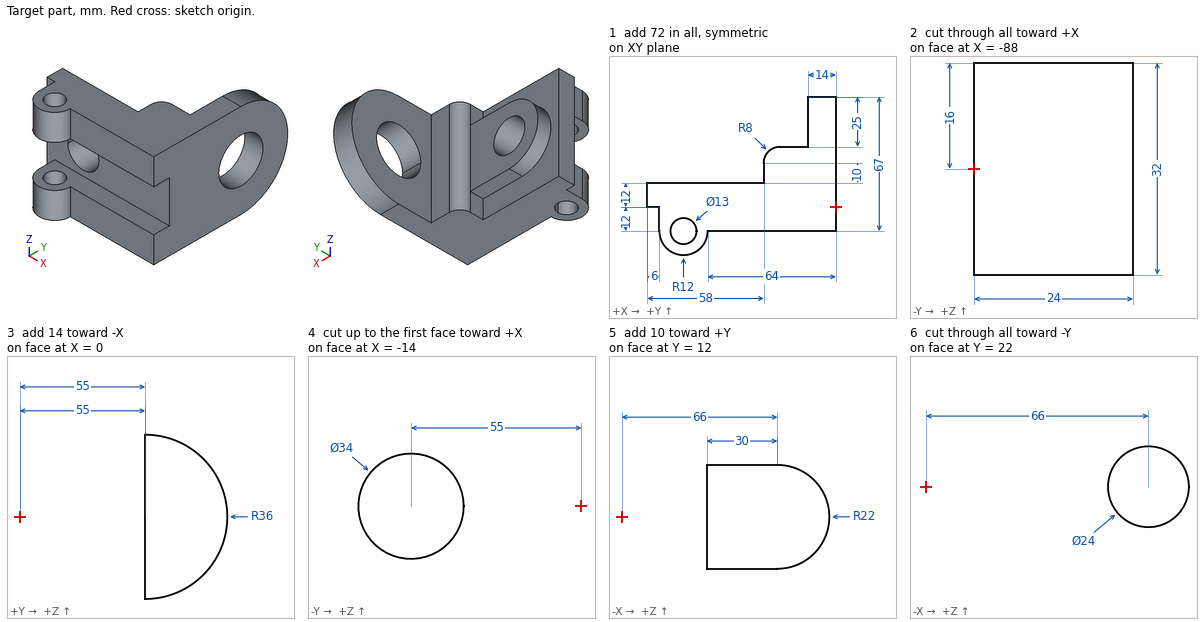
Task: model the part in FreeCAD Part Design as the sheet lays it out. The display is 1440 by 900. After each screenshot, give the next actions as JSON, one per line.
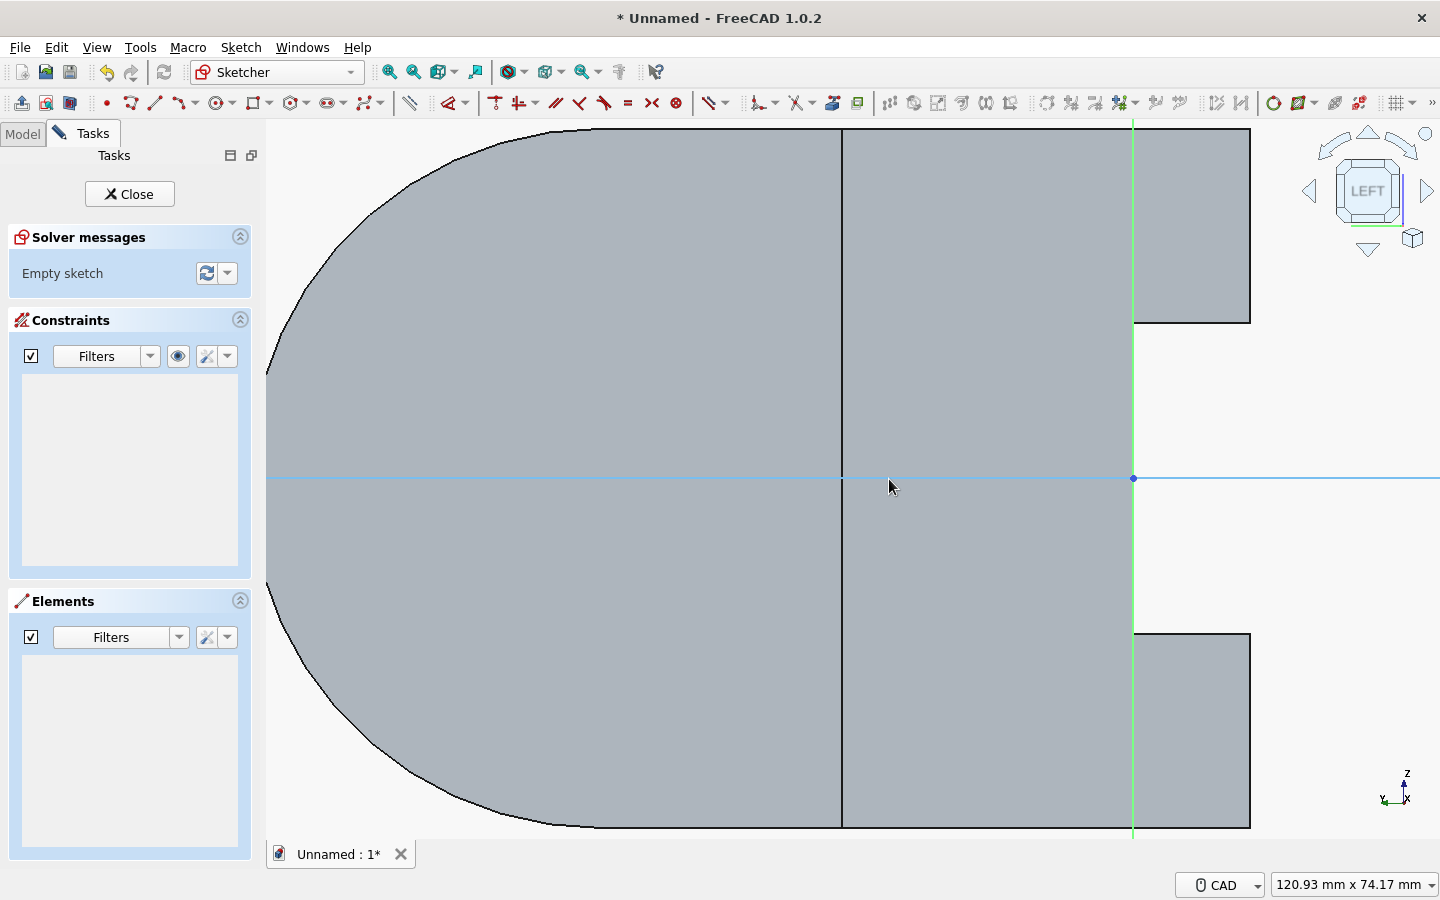
{"action": "left_click", "coordinate": [216, 104]}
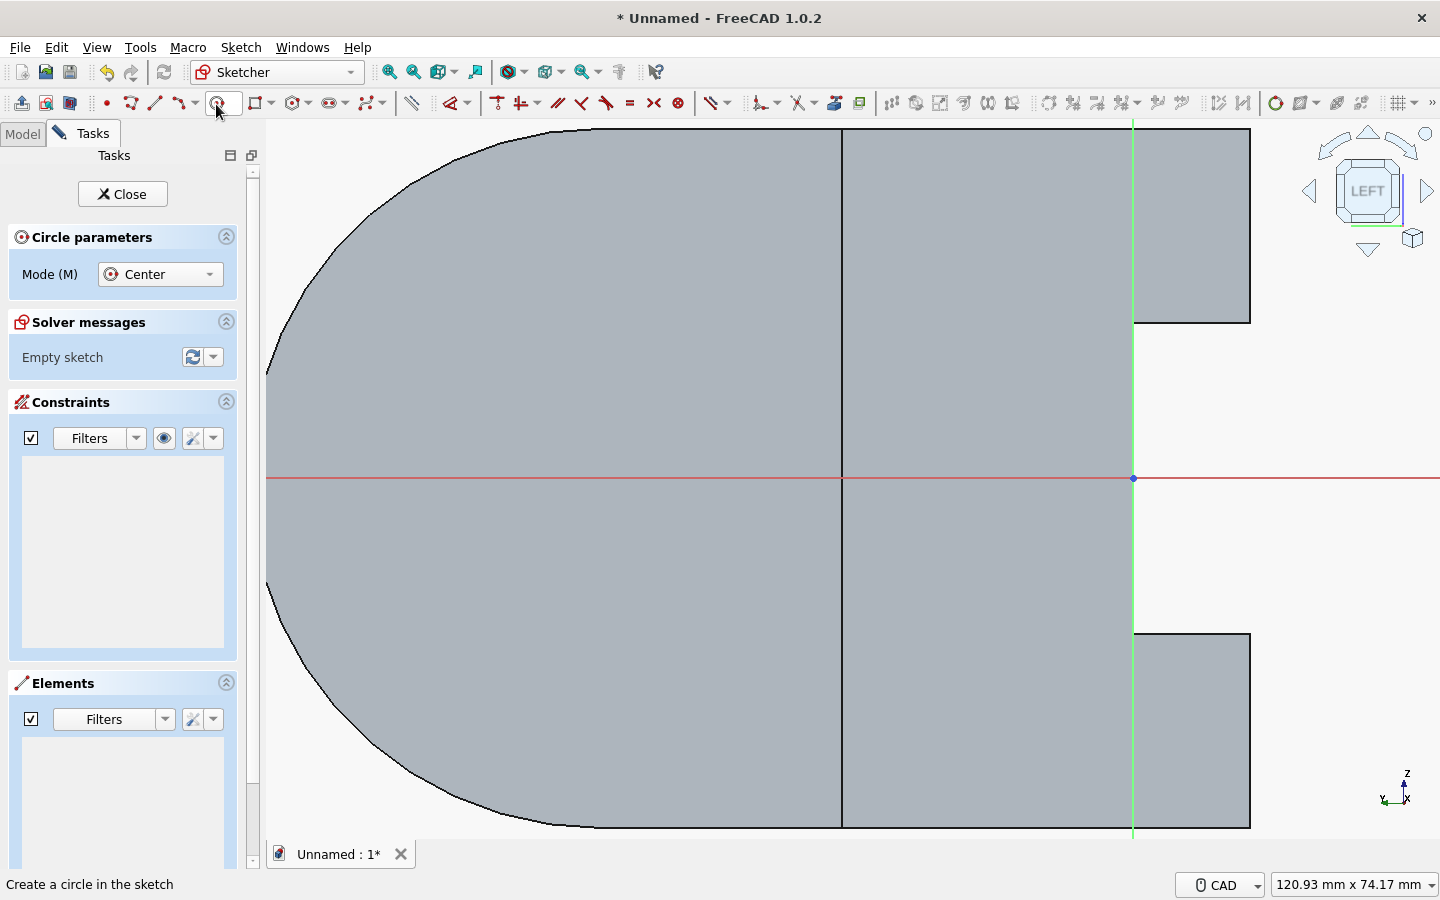
{"action": "left_click", "coordinate": [600, 478]}
{"action": "mouse_move", "coordinate": [716, 362]}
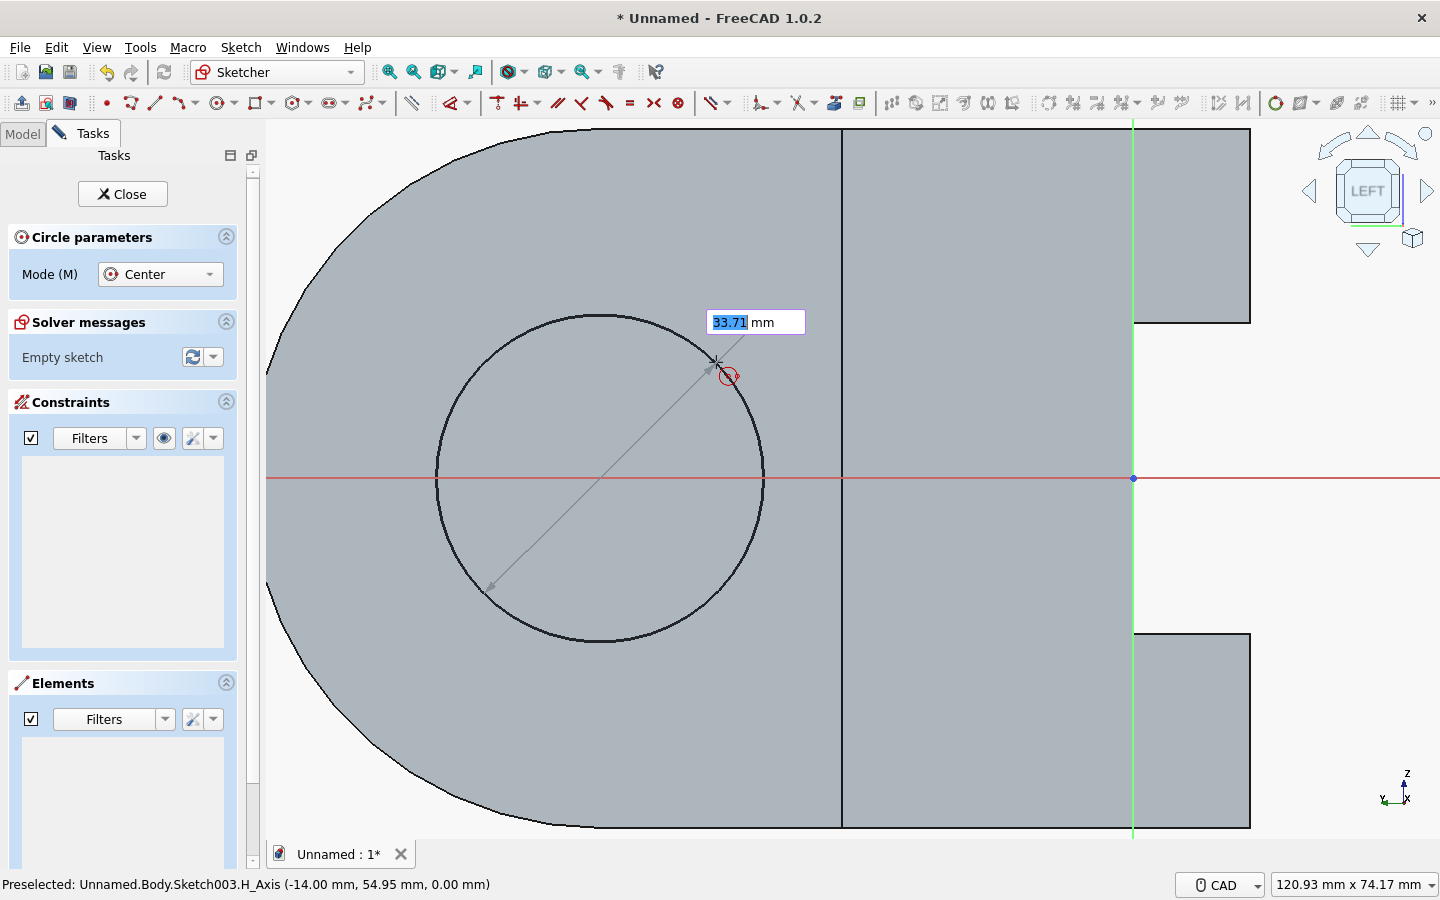
{"action": "type", "text": "34"}
{"action": "key", "text": "Return"}
{"action": "key", "text": "Escape"}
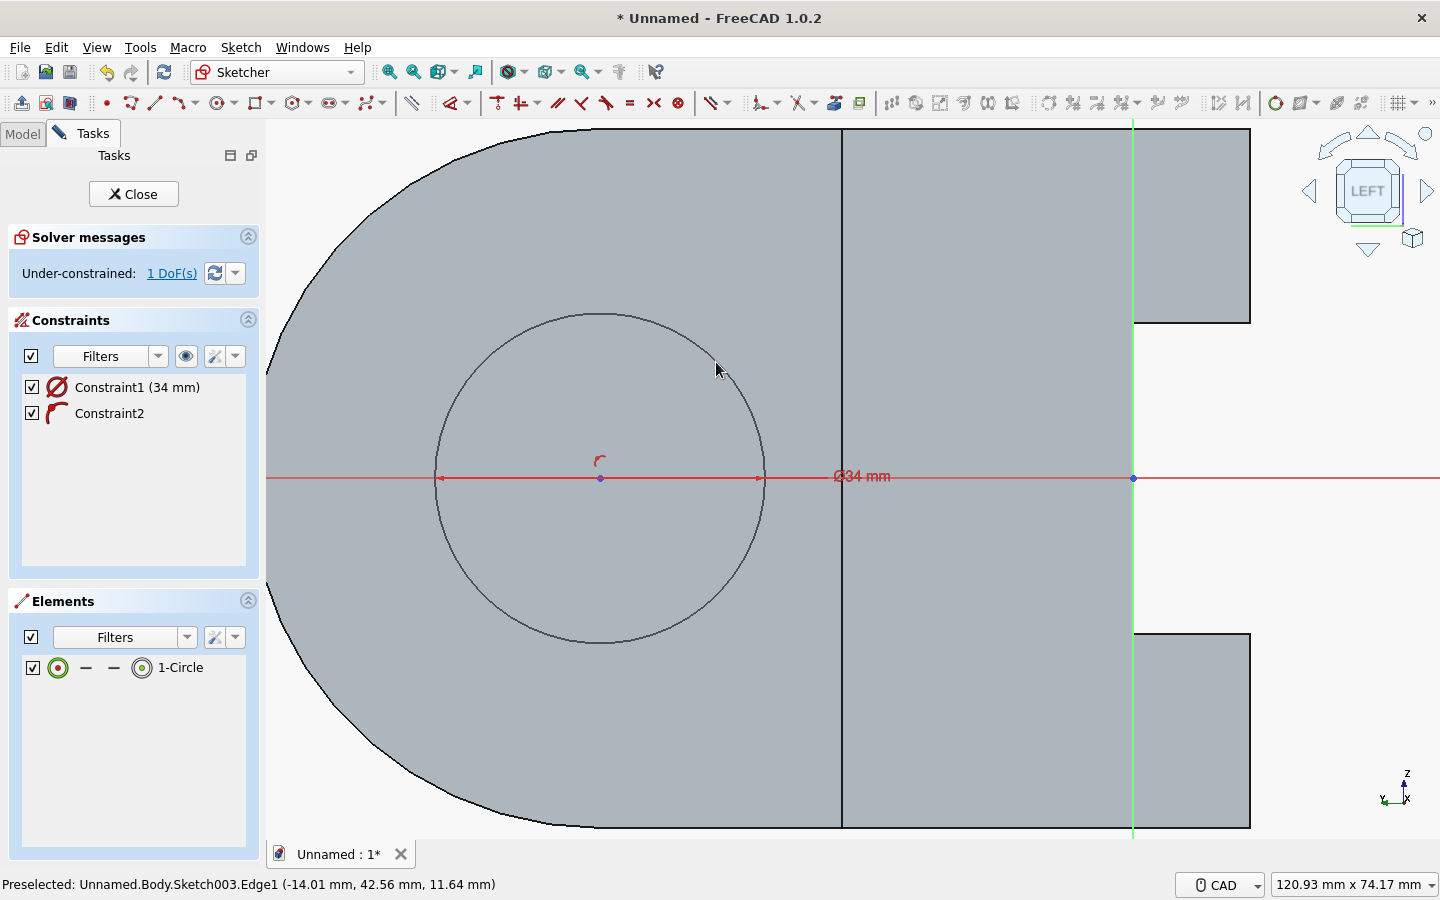
{"action": "left_click", "coordinate": [450, 104]}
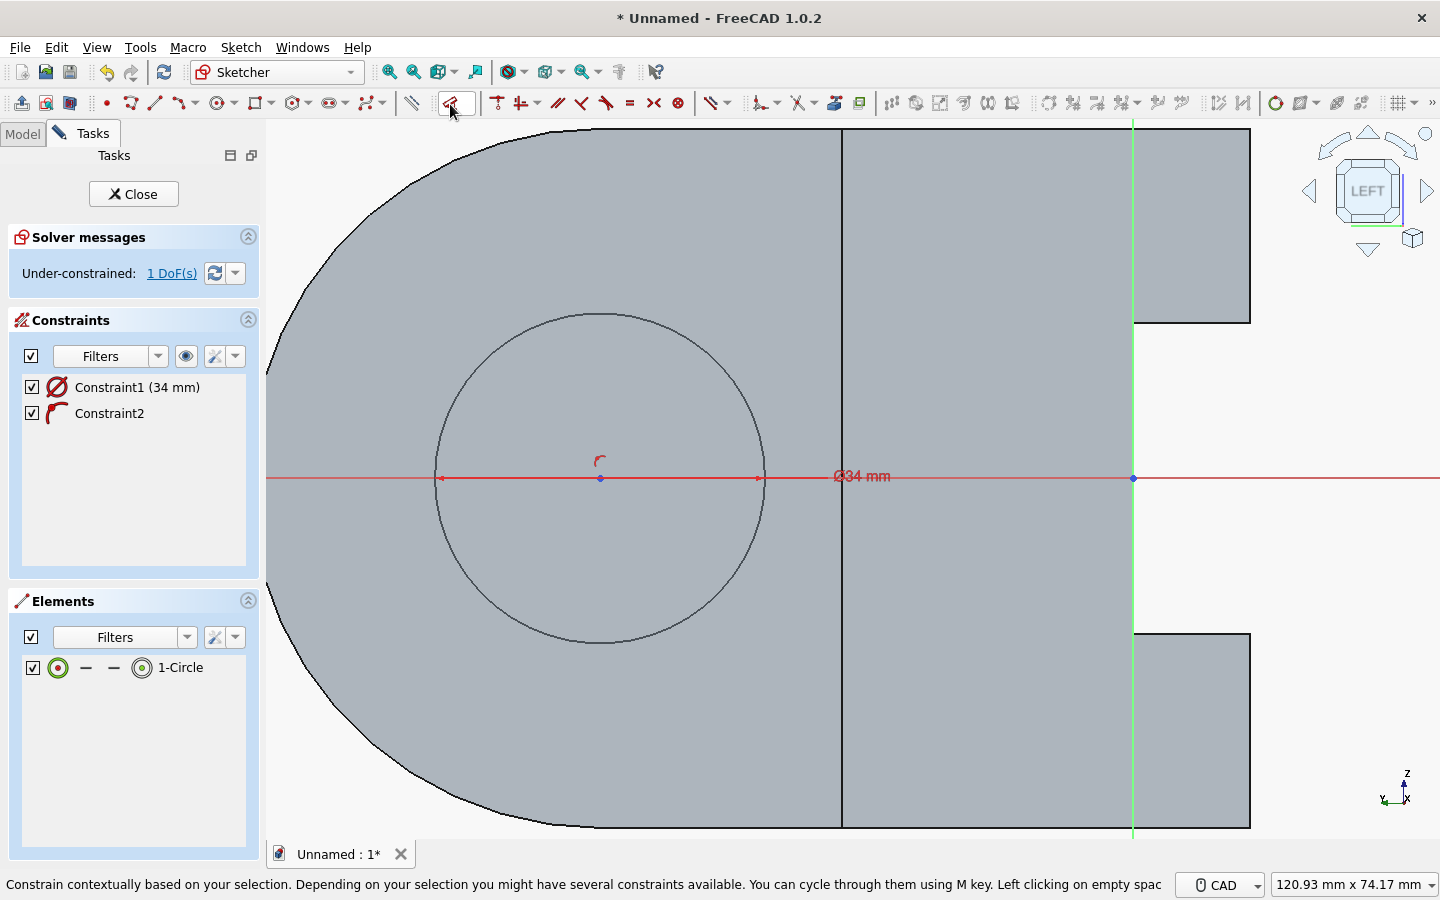
{"action": "left_click", "coordinate": [600, 478]}
{"action": "left_click", "coordinate": [867, 512]}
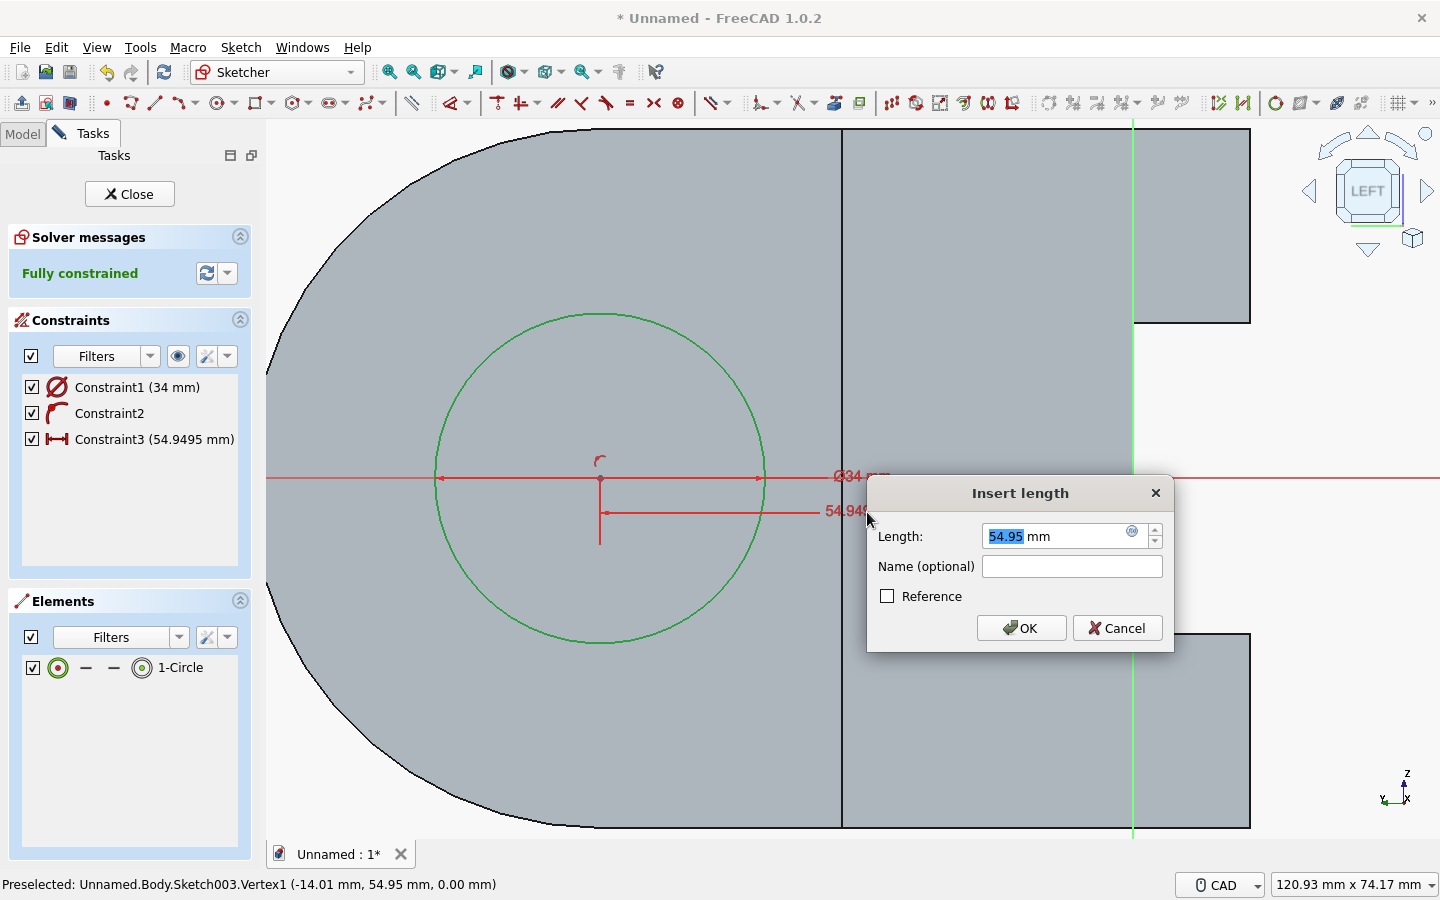
{"action": "type", "text": "55"}
{"action": "key", "text": "Return"}
{"action": "key", "text": "Escape"}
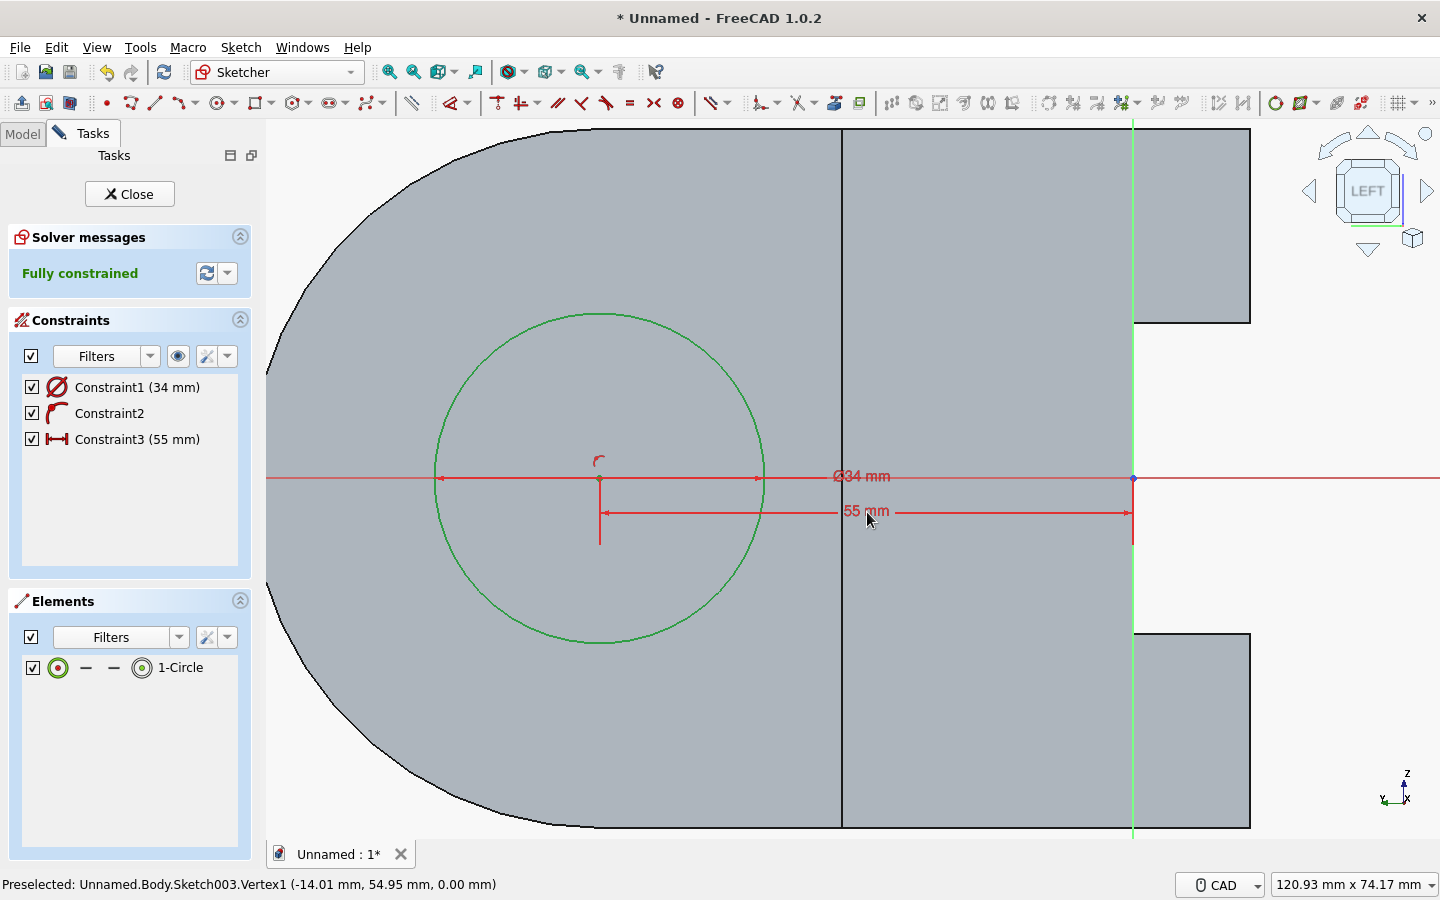
{"action": "left_click", "coordinate": [130, 194]}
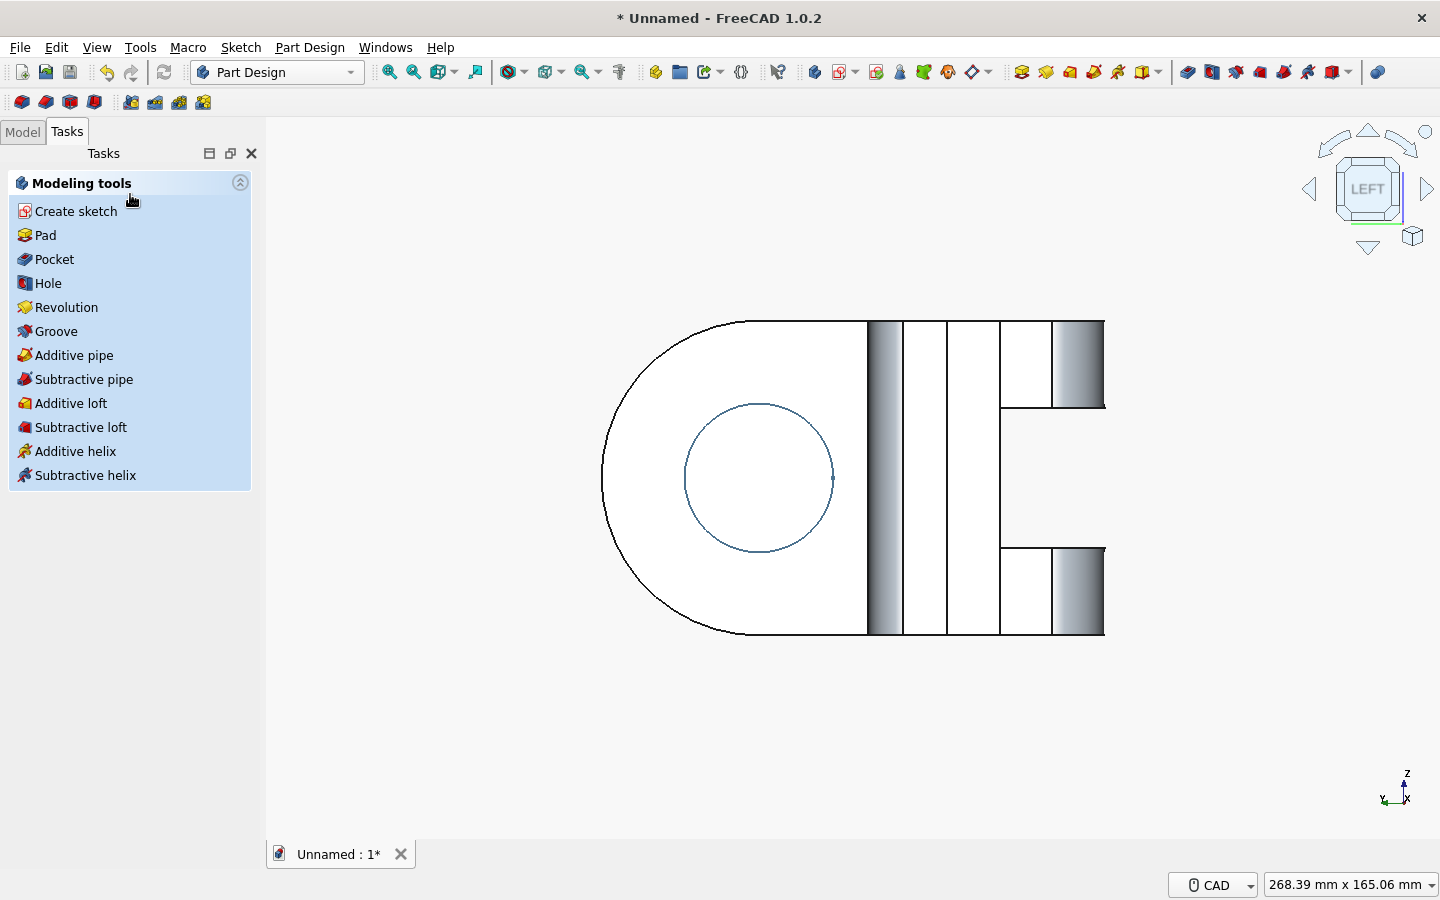
{"action": "left_click", "coordinate": [1188, 72]}